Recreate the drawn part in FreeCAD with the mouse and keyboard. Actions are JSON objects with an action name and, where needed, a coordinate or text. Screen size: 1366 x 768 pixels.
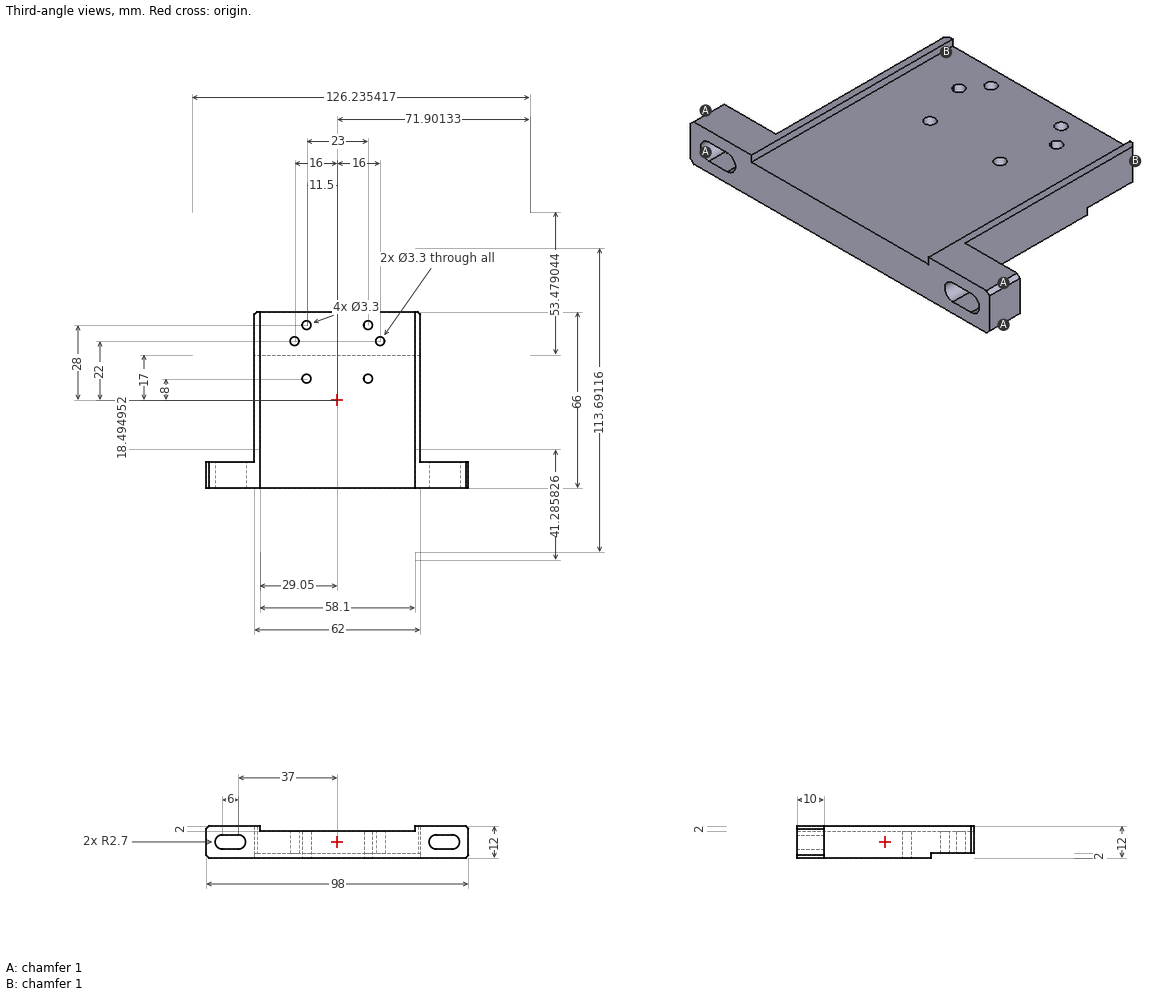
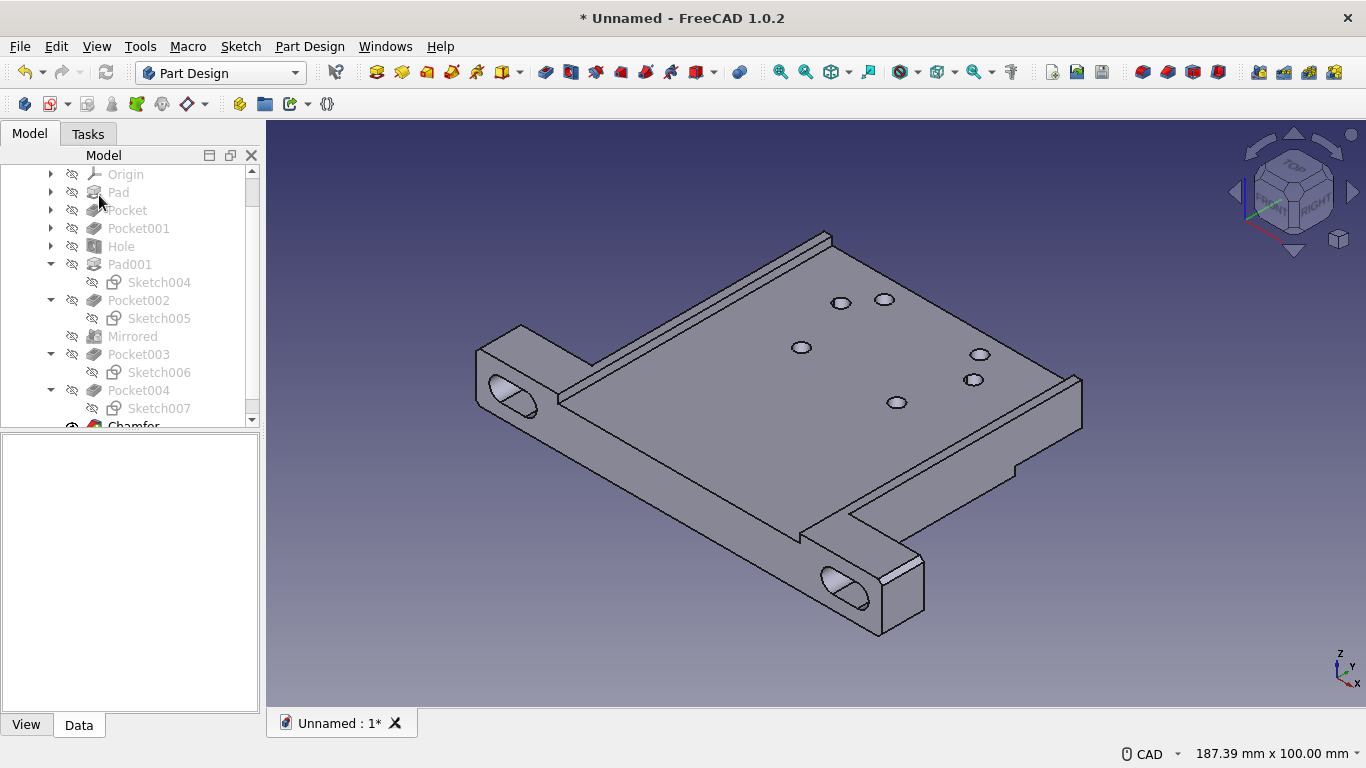
{"action": "key", "text": "2"}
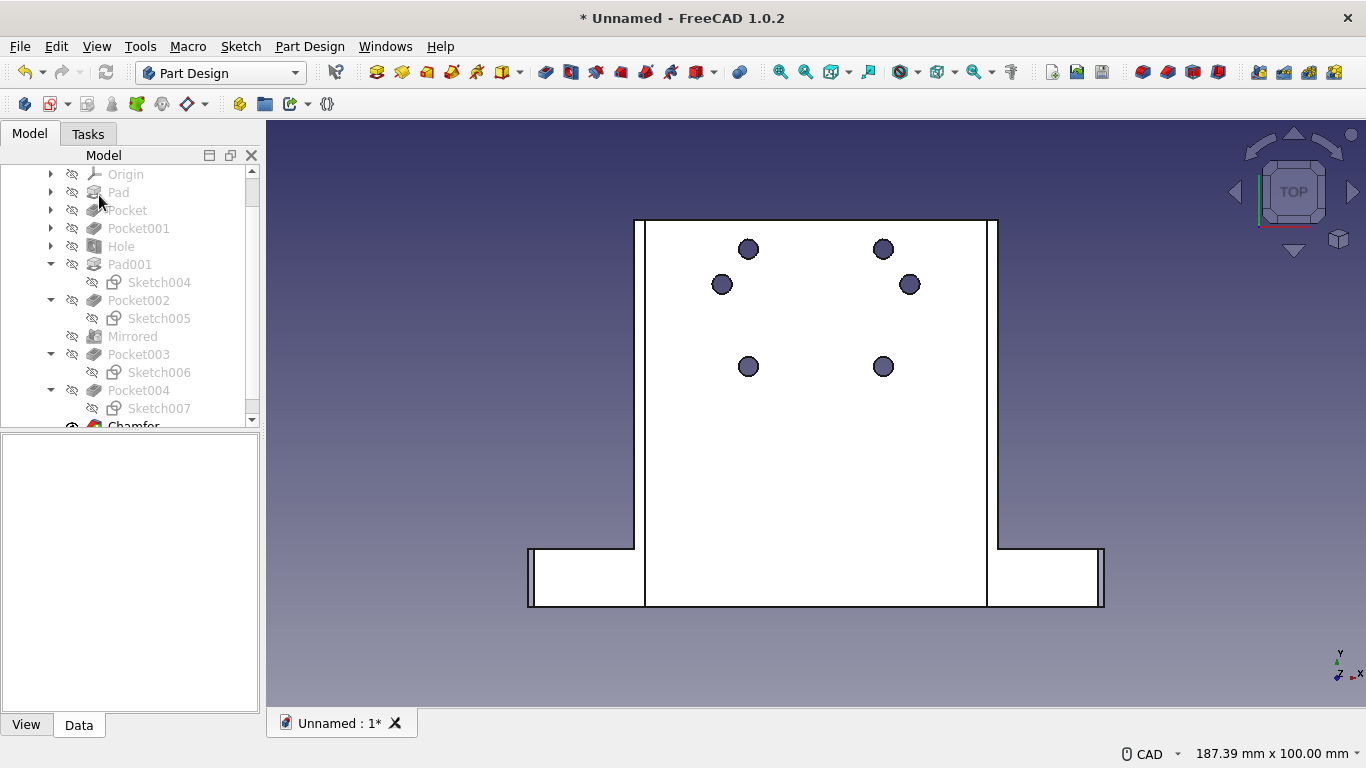
{"action": "key", "text": "1"}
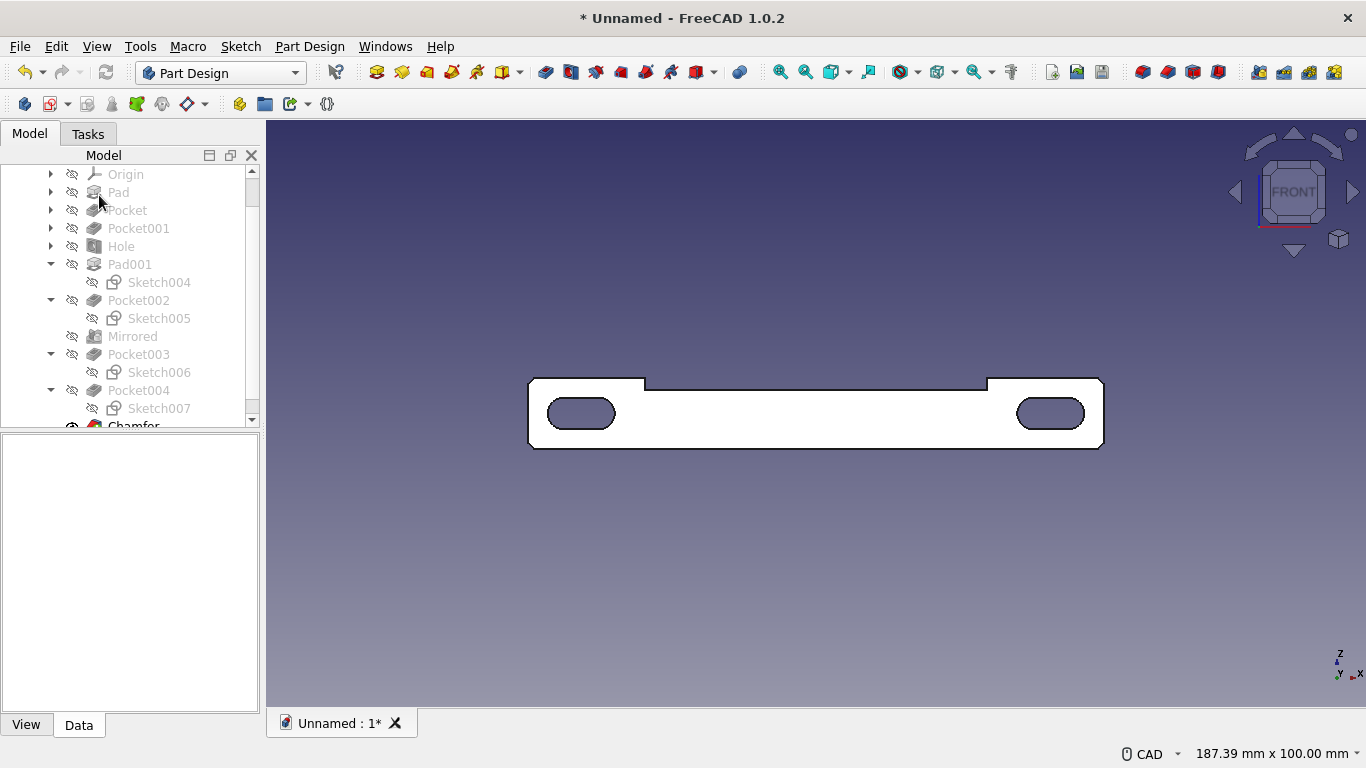
{"action": "key", "text": "3"}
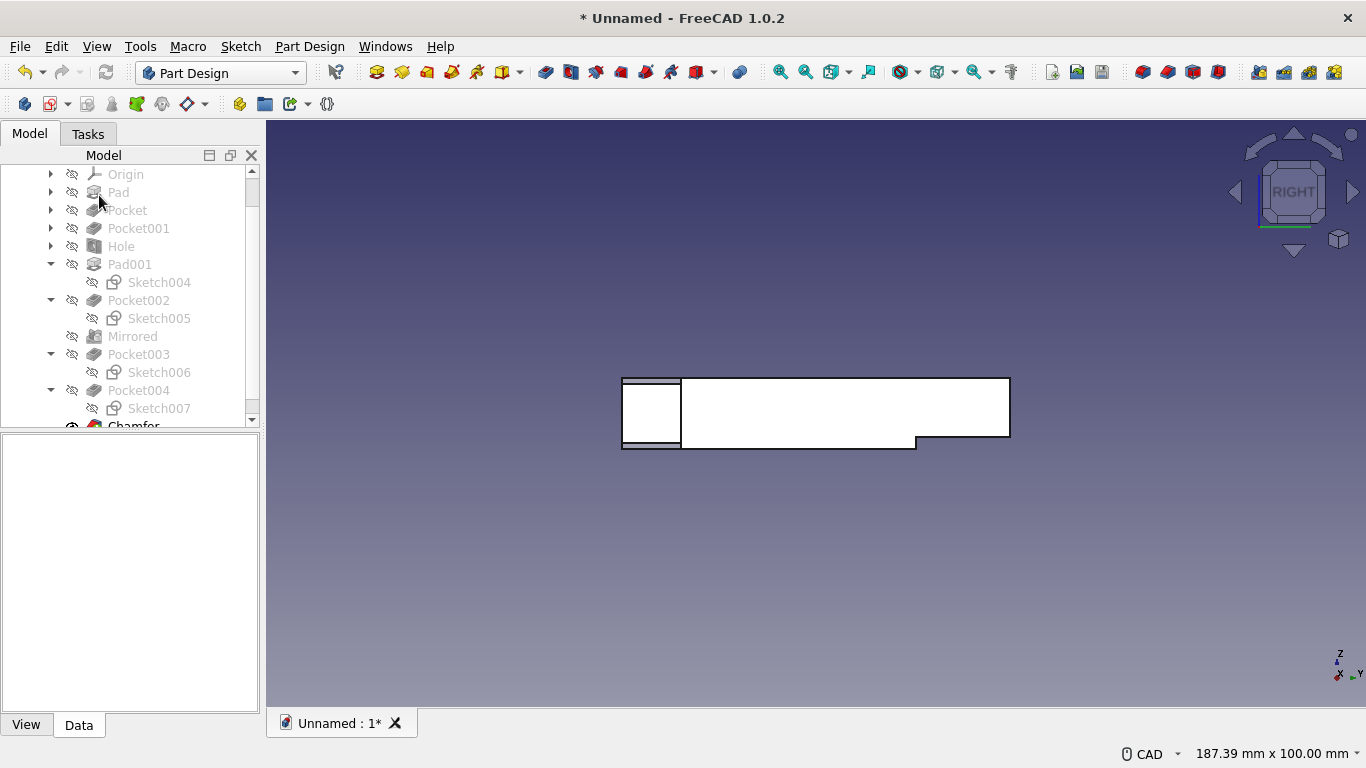
{"action": "left_click", "coordinate": [781, 72]}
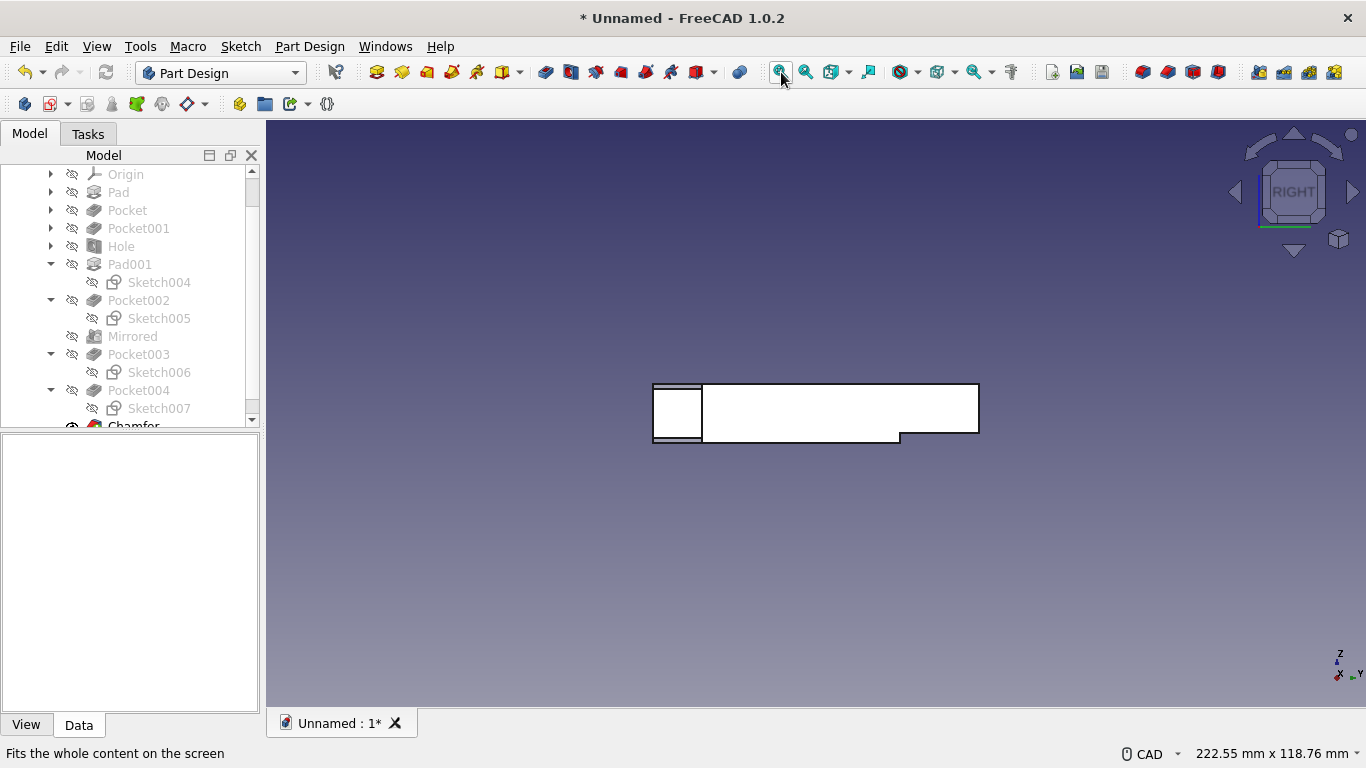
{"action": "left_click", "coordinate": [979, 408]}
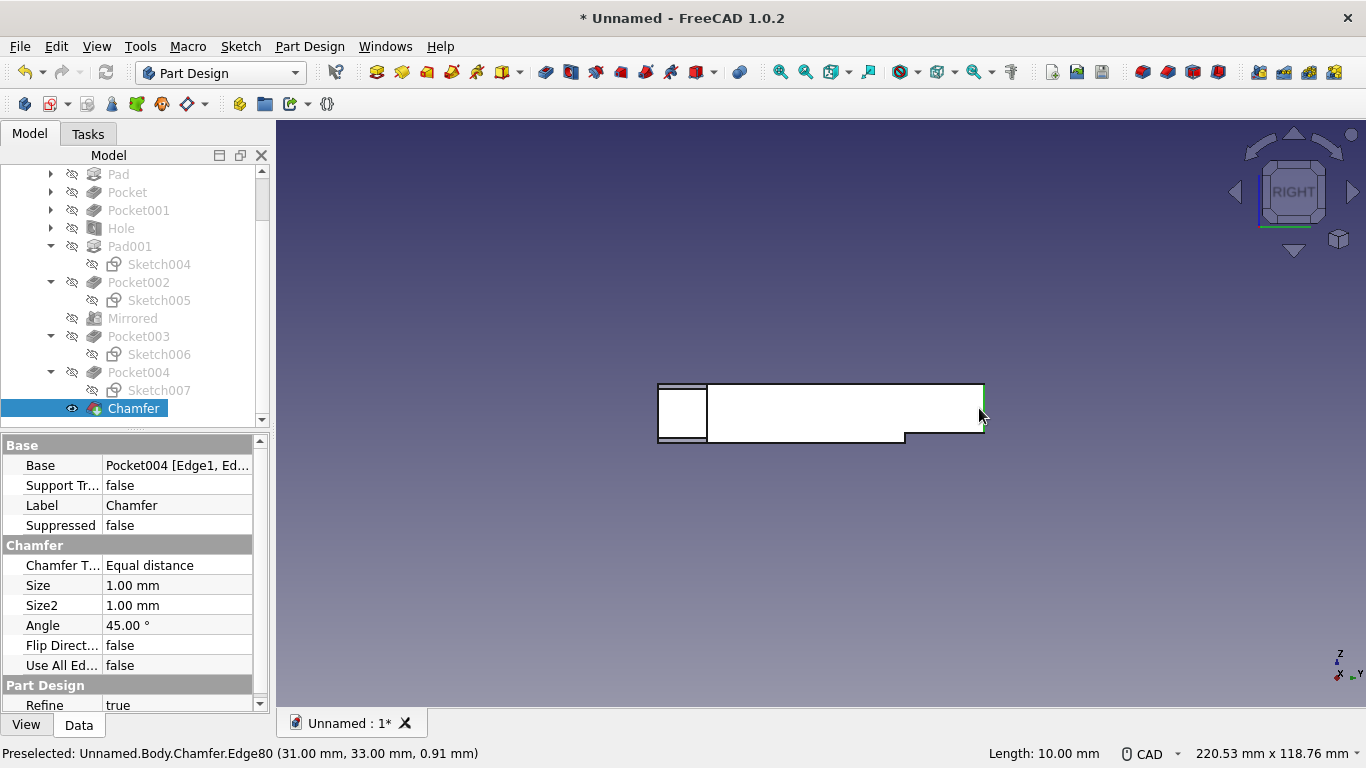
{"action": "key", "text": "5"}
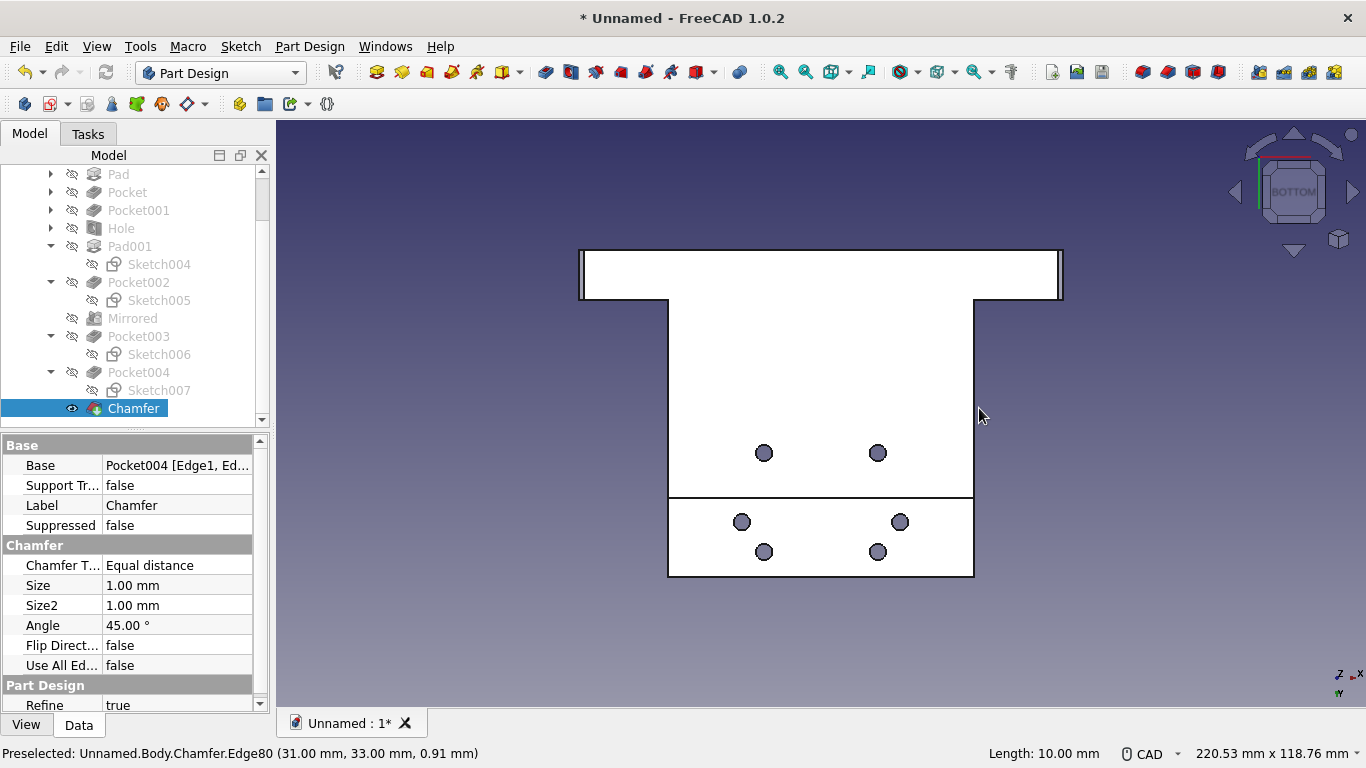
{"action": "key", "text": "4"}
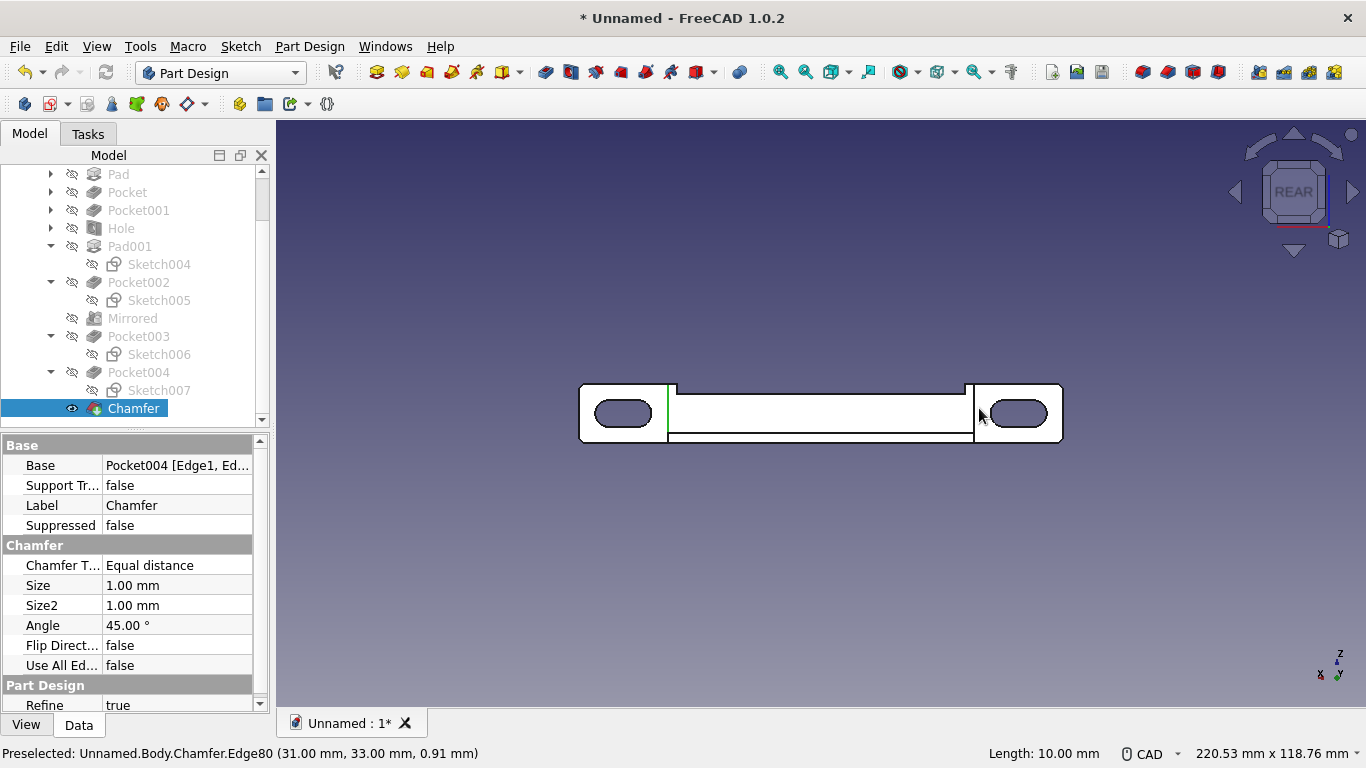
{"action": "left_click", "coordinate": [781, 72]}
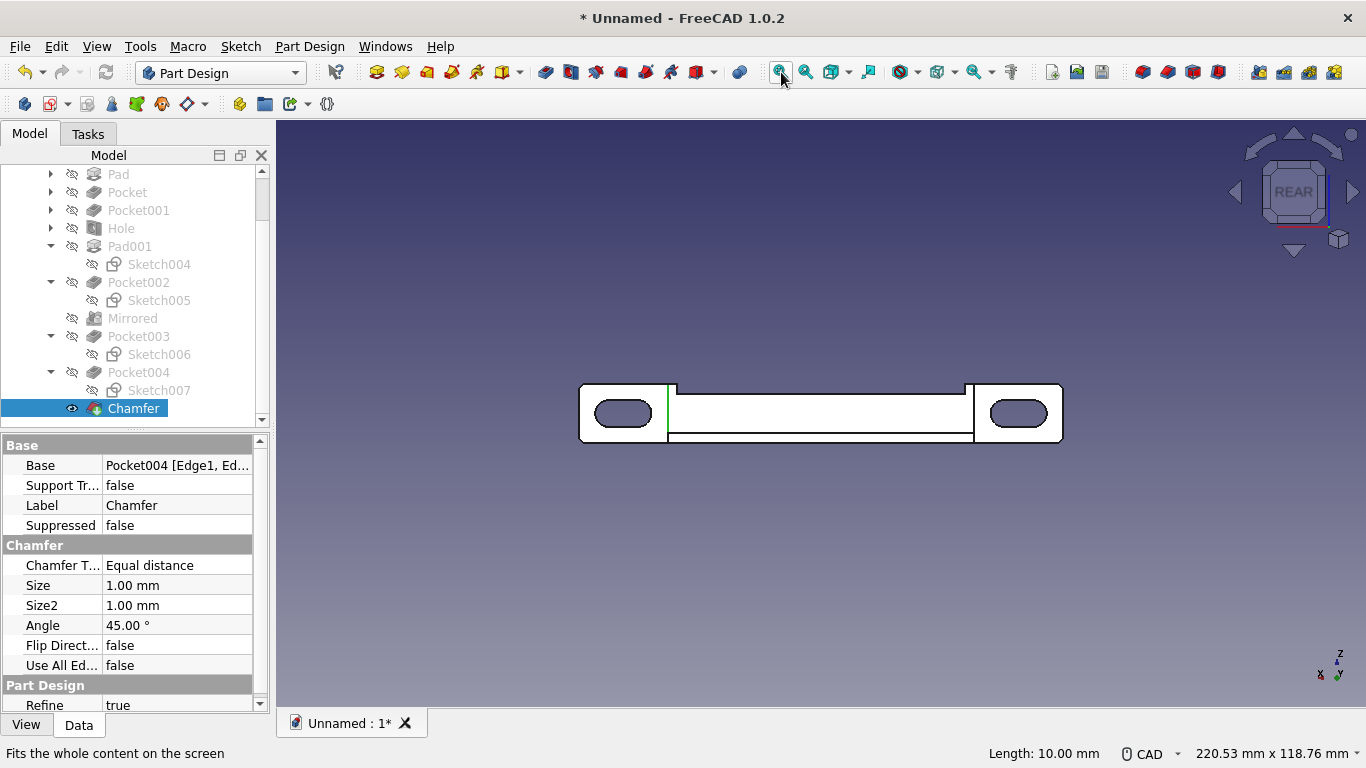
{"action": "left_click", "coordinate": [974, 408], "text": "ctrl"}